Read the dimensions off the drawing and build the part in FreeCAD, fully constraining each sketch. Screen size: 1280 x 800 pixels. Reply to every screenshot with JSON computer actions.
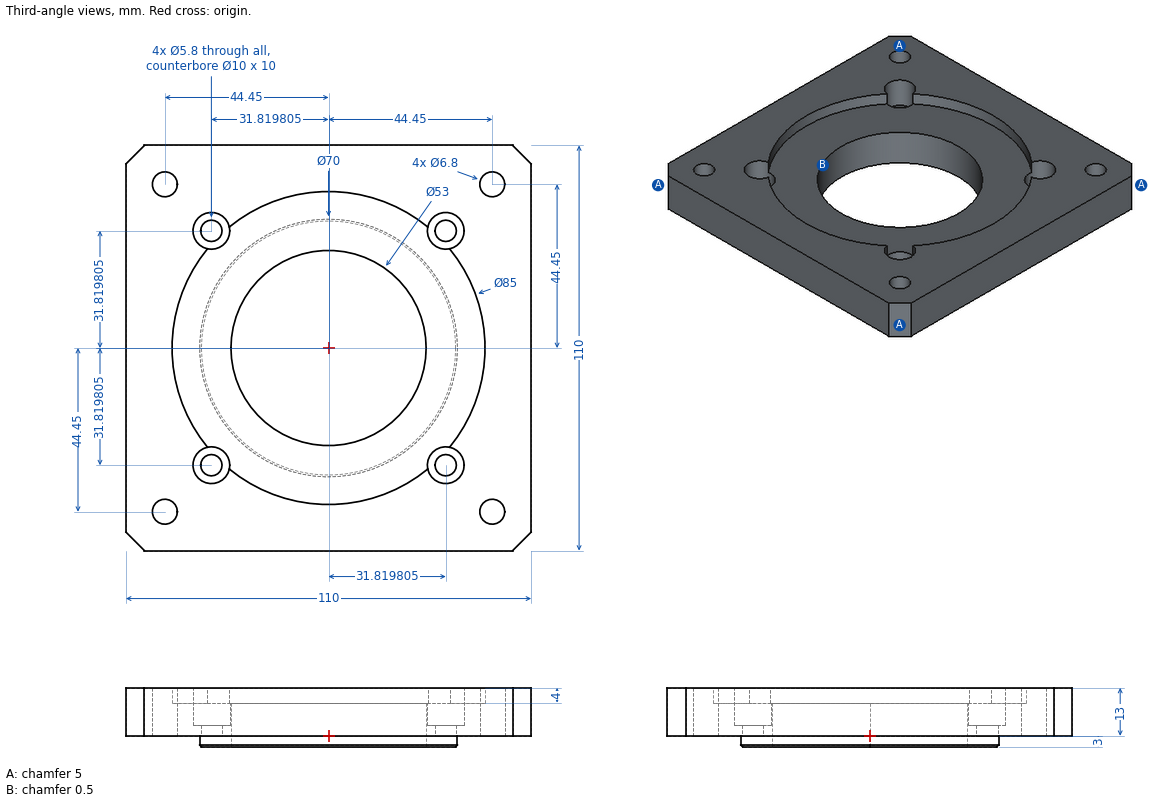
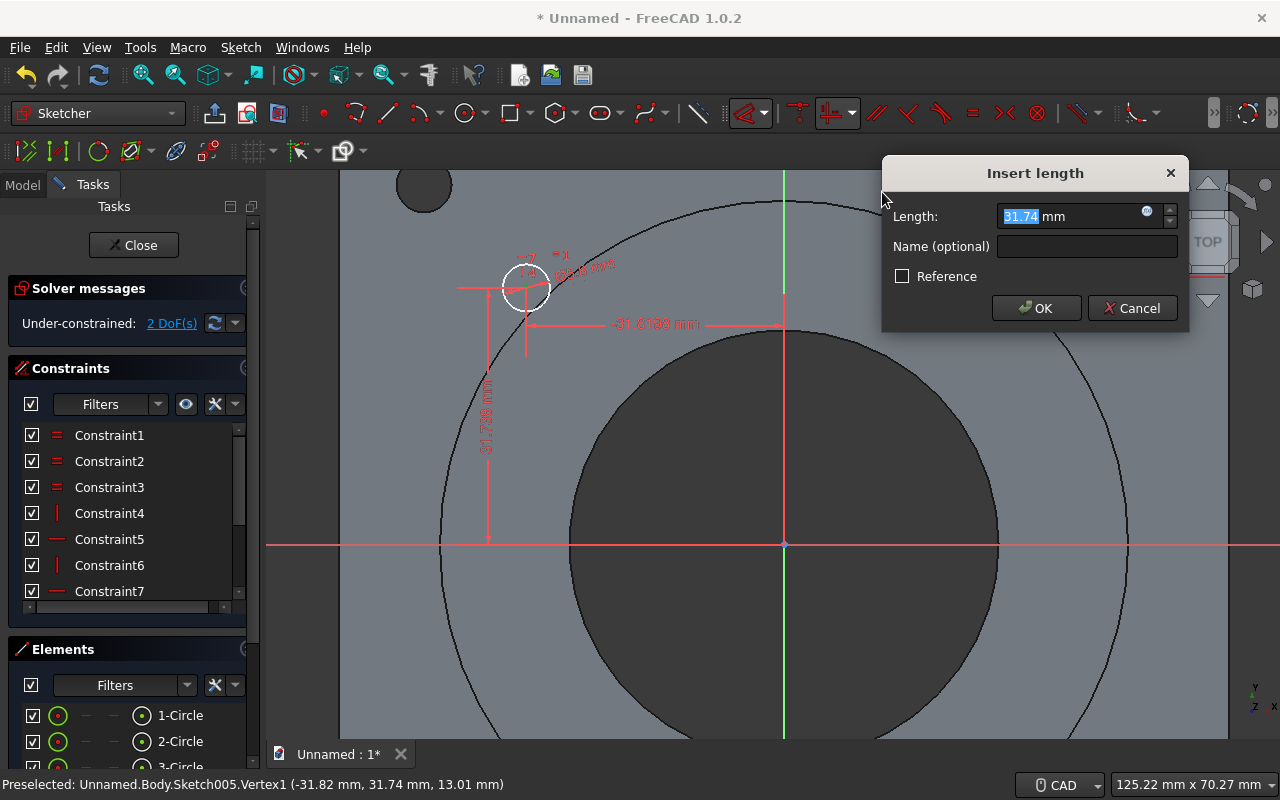
{"action": "type", "text": "31.819805"}
{"action": "key", "text": "Return"}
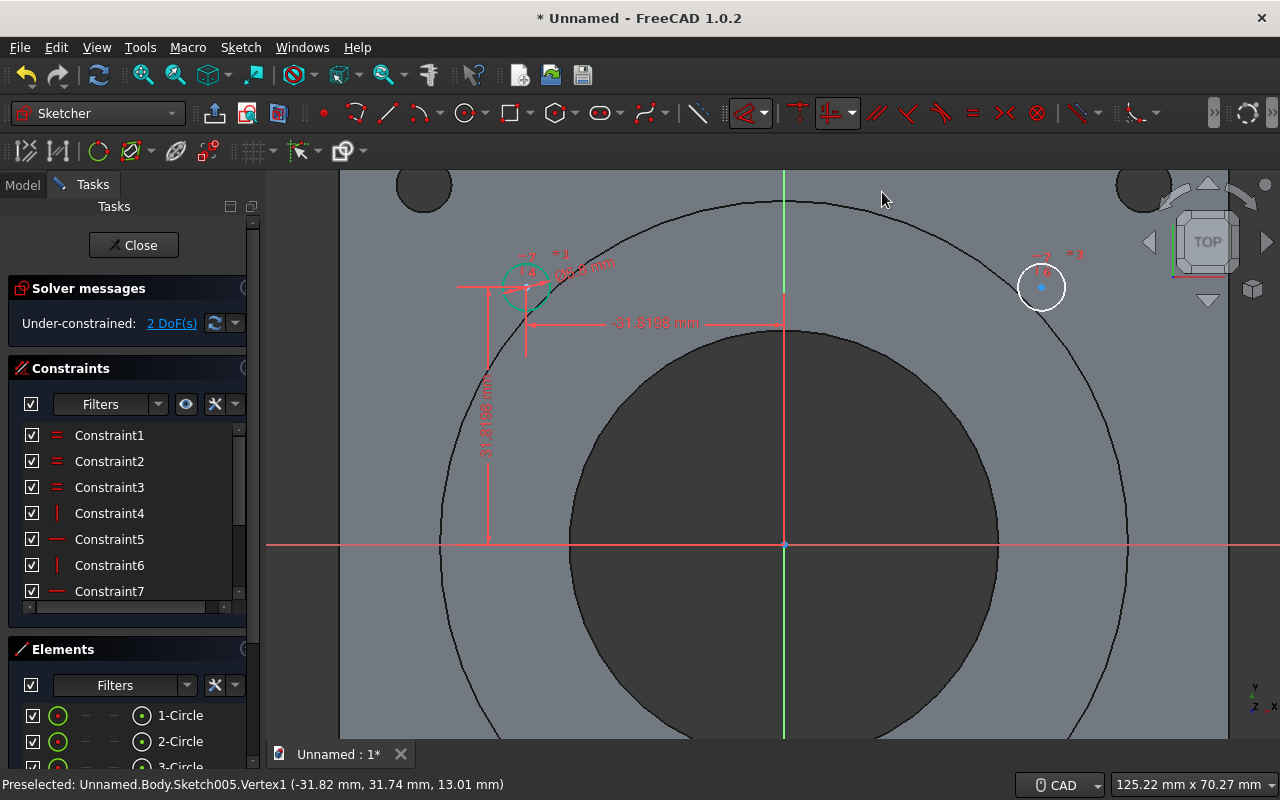
{"action": "scroll", "coordinate": [543, 271], "scroll_direction": "down", "scroll_amount": 2}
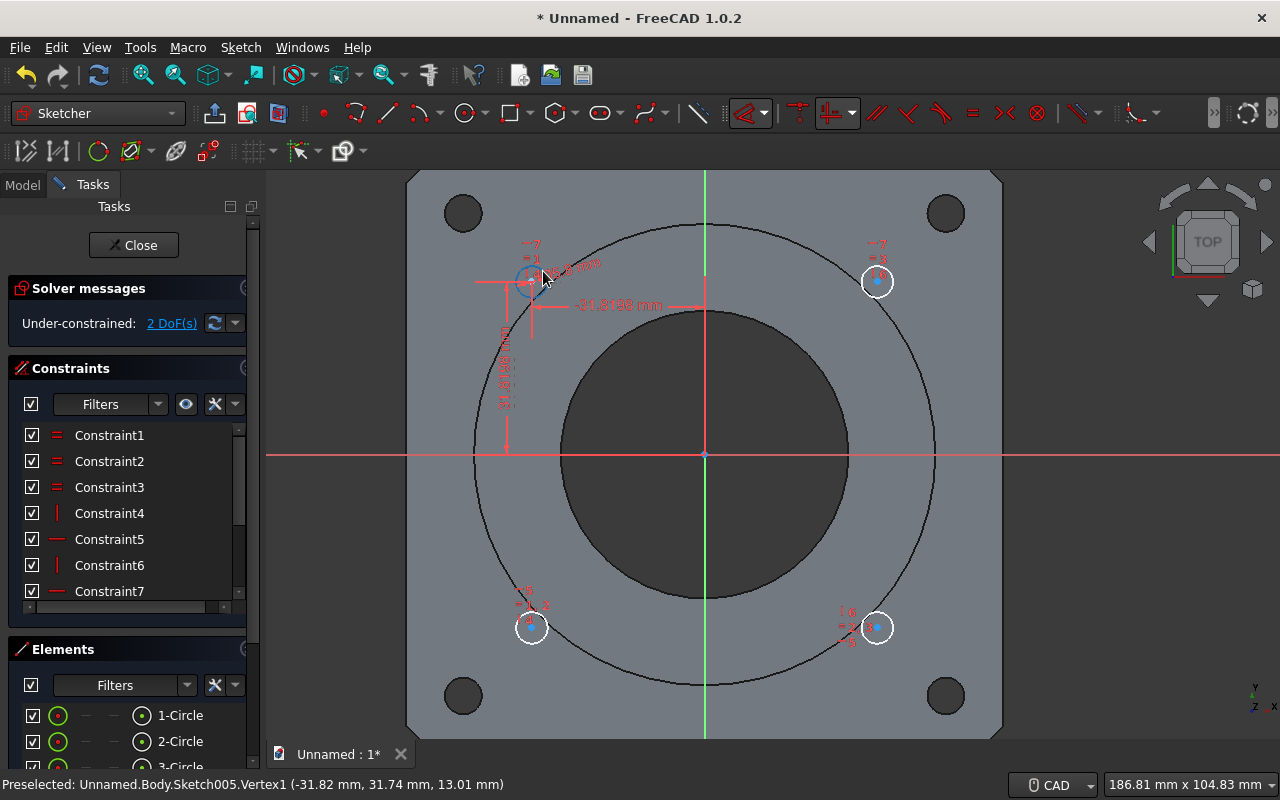
{"action": "left_click", "coordinate": [532, 628]}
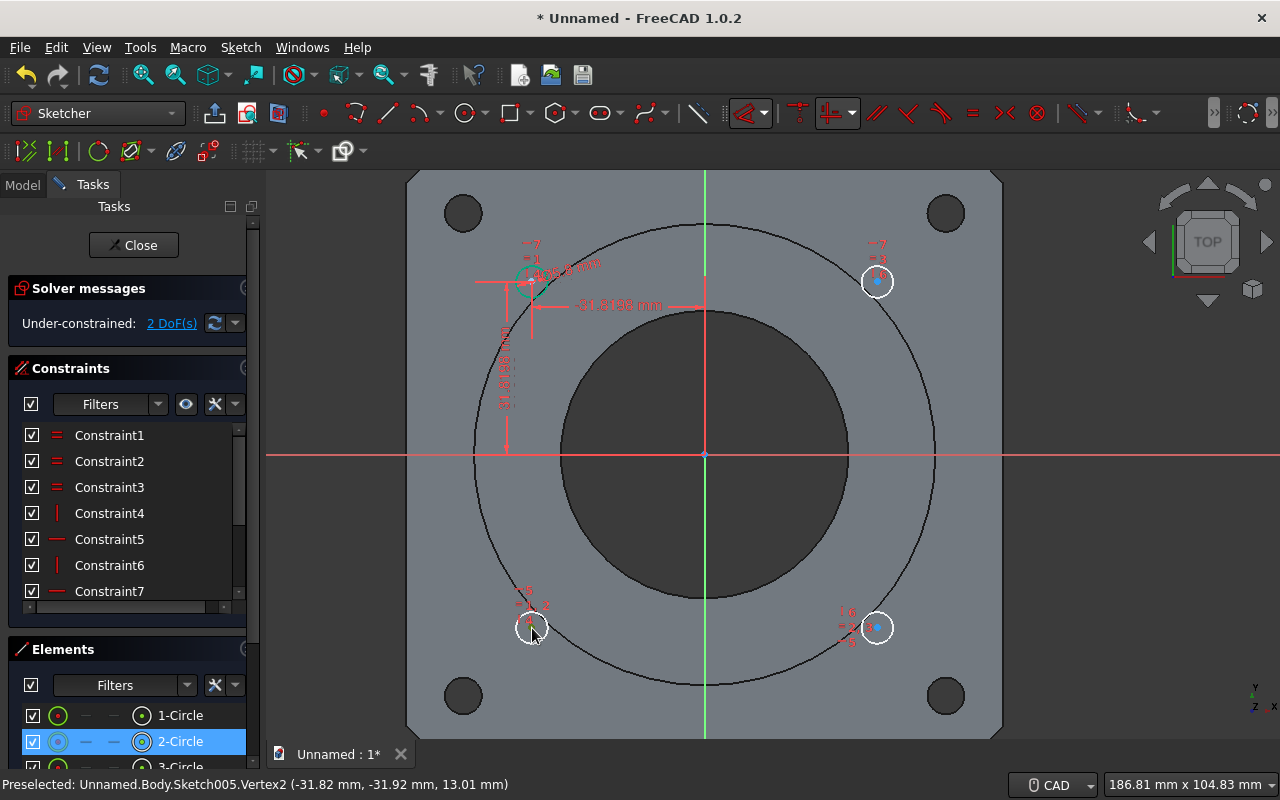
{"action": "left_click", "coordinate": [766, 114]}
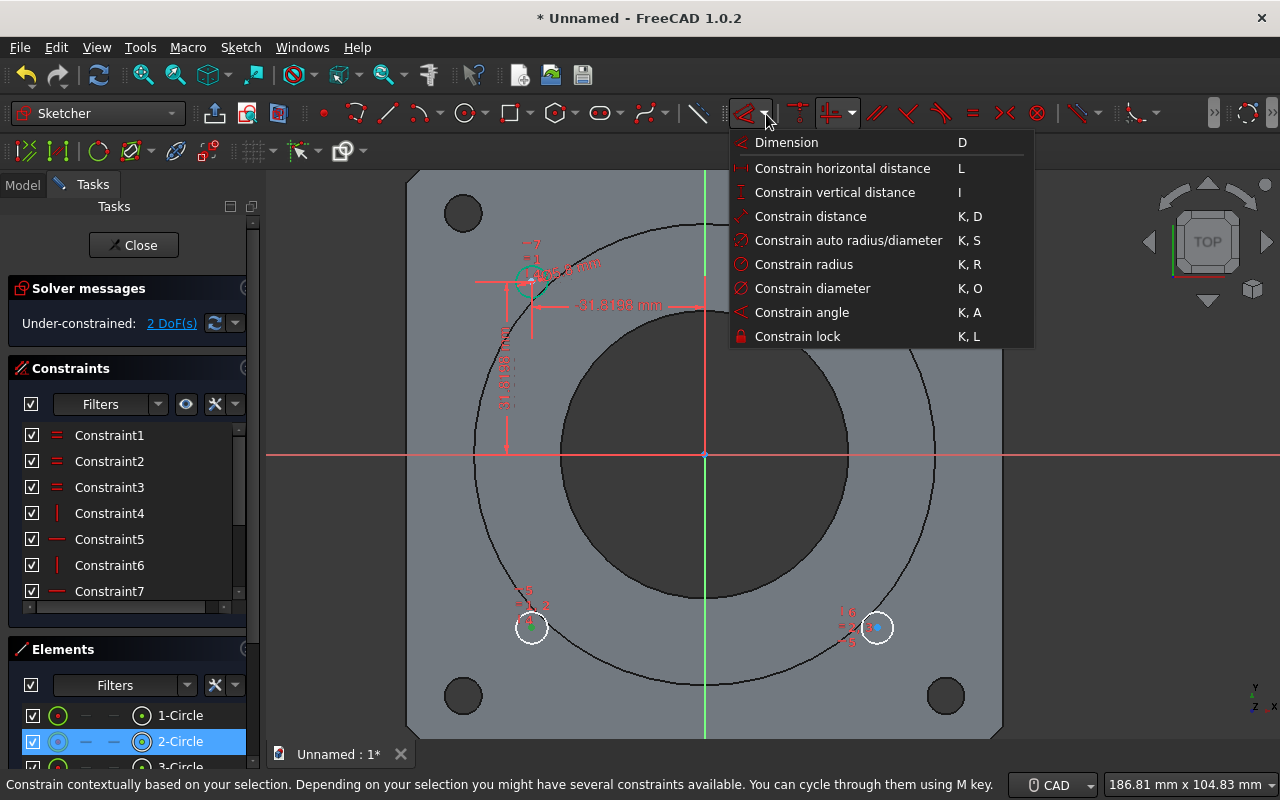
{"action": "left_click", "coordinate": [882, 192]}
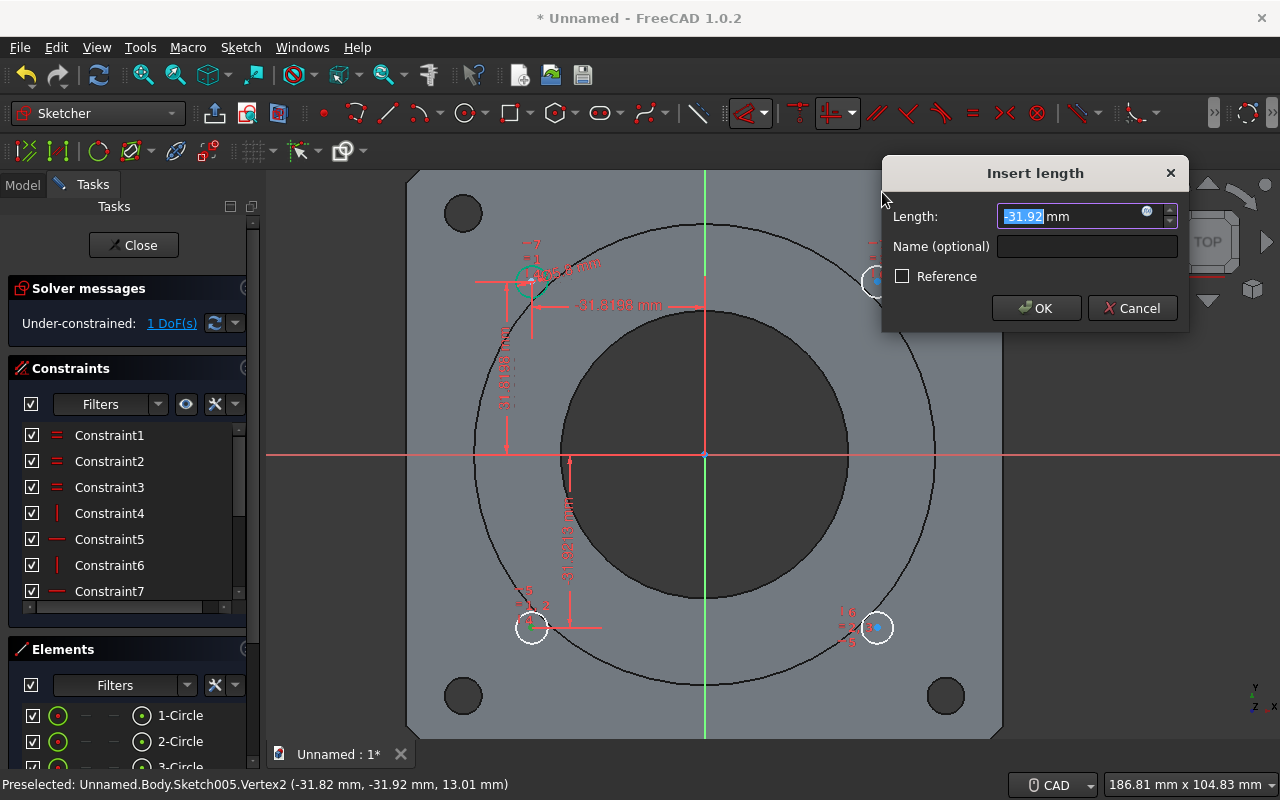
{"action": "type", "text": "-31.819805"}
{"action": "key", "text": "Return"}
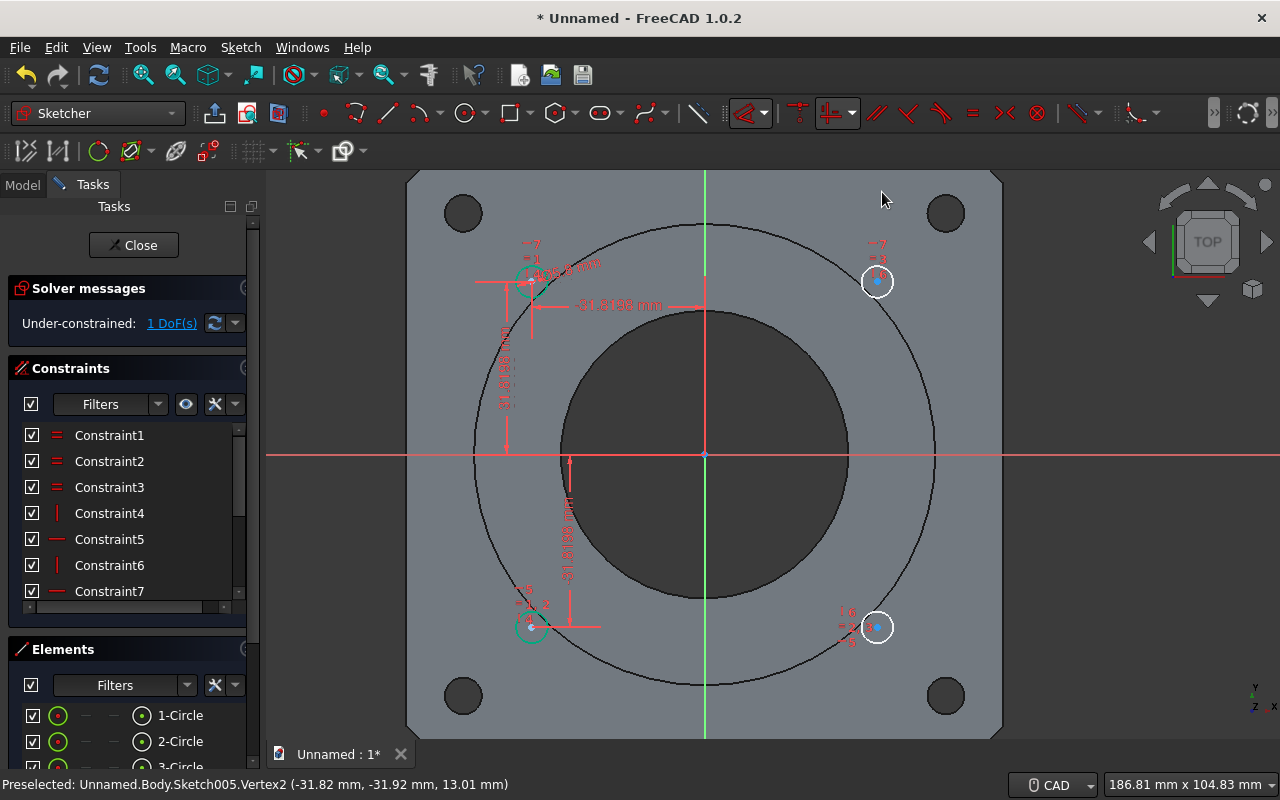
{"action": "left_click", "coordinate": [877, 627]}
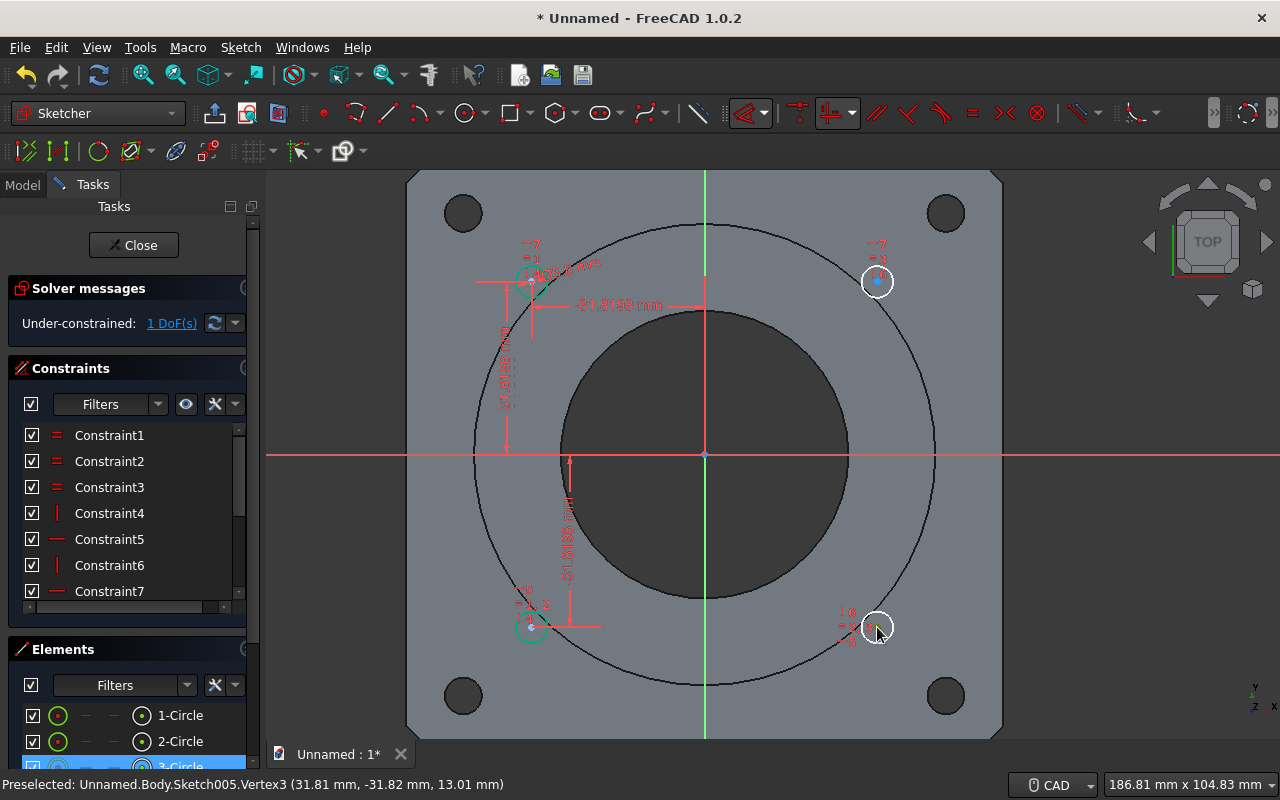
{"action": "key", "text": "l"}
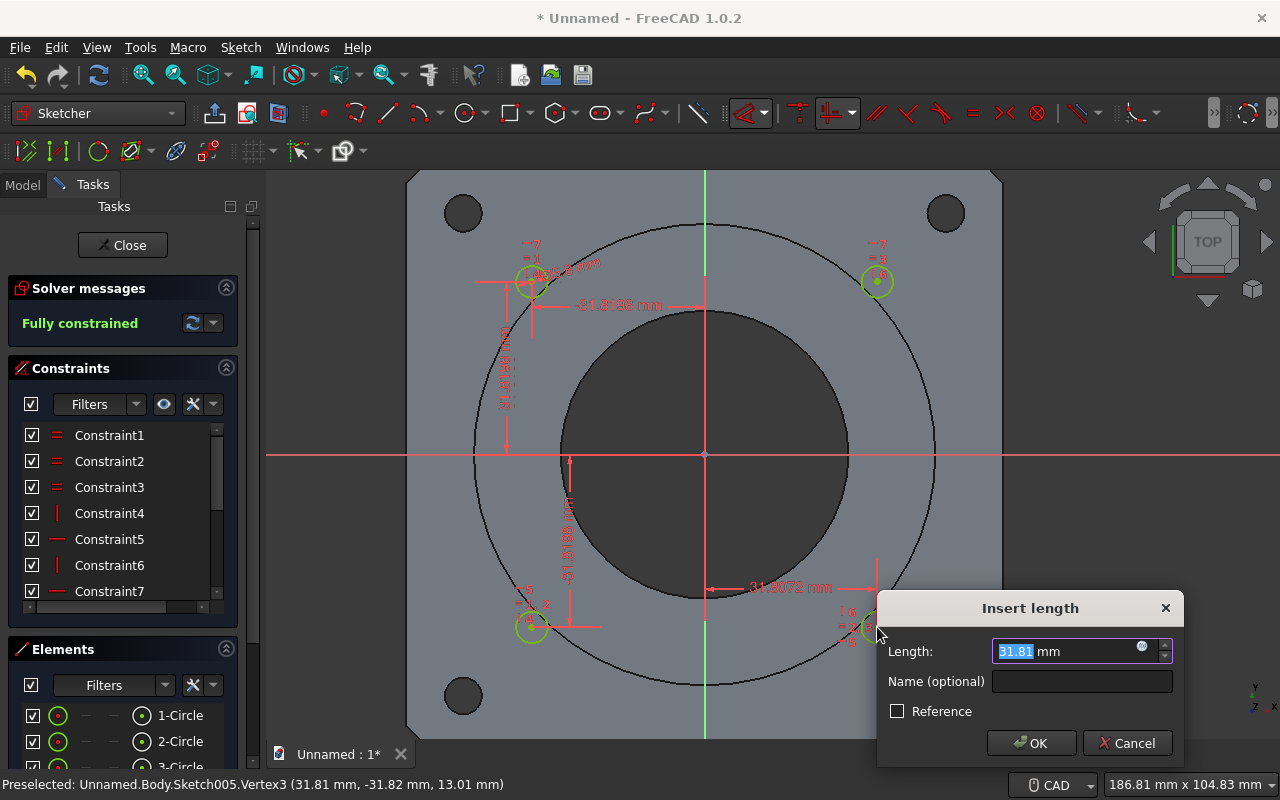
{"action": "type", "text": "31.819805"}
{"action": "key", "text": "Return"}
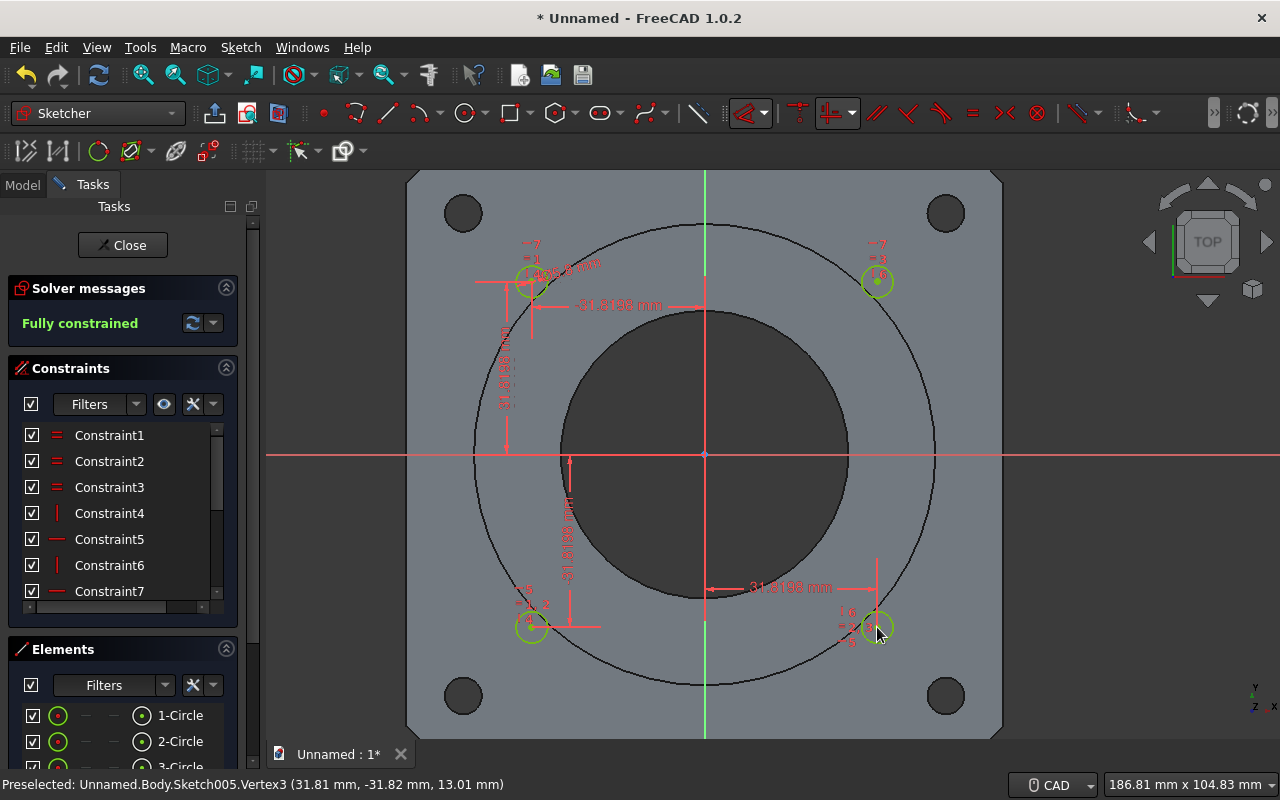
{"action": "left_click", "coordinate": [123, 245]}